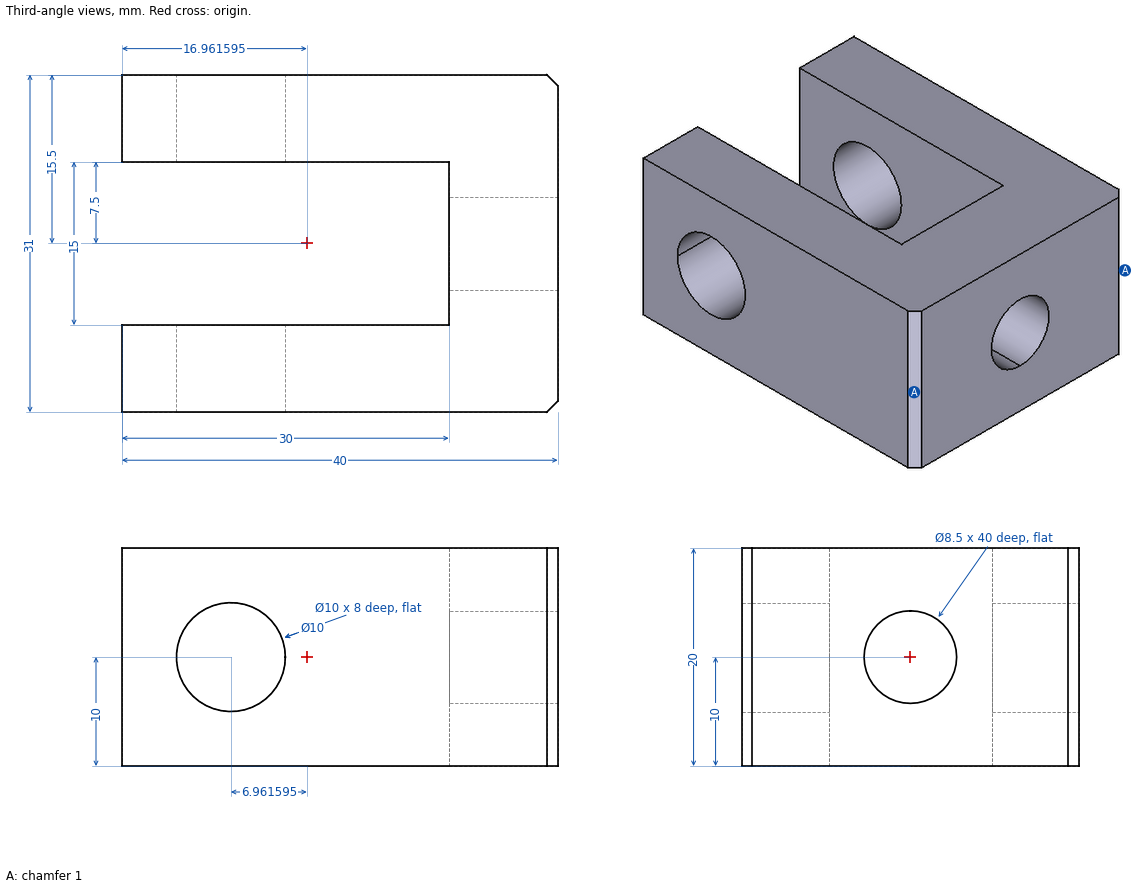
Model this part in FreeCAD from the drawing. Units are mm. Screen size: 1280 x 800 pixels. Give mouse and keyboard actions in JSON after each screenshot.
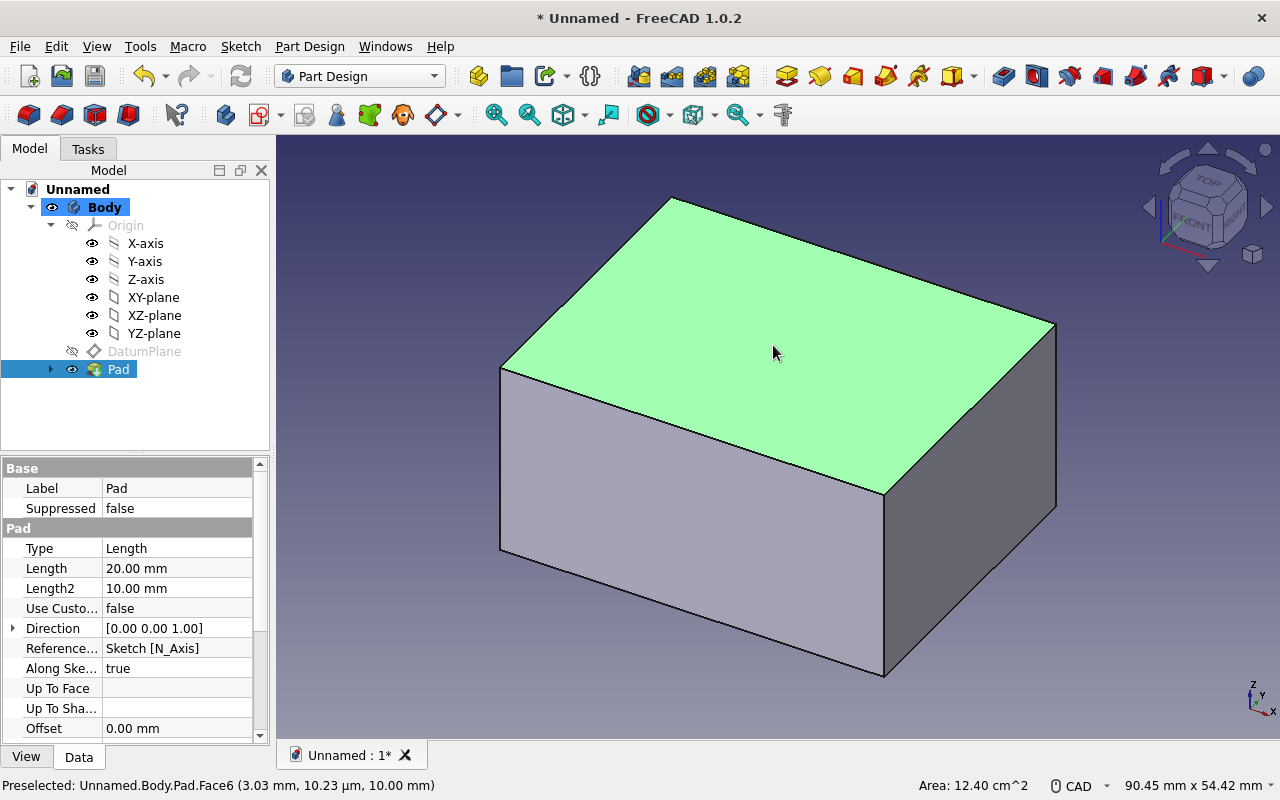
{"action": "left_click", "coordinate": [258, 116]}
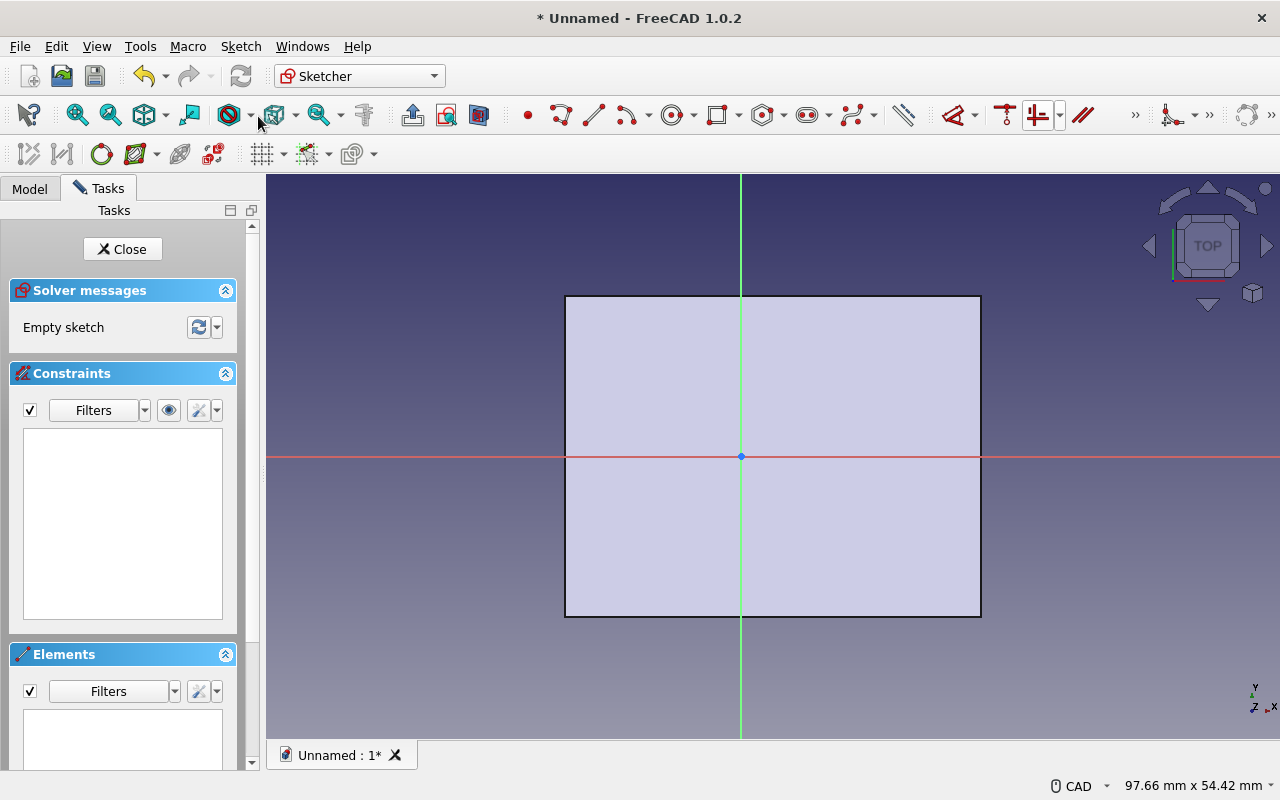
{"action": "scroll", "coordinate": [741, 456], "scroll_direction": "up", "scroll_amount": 3}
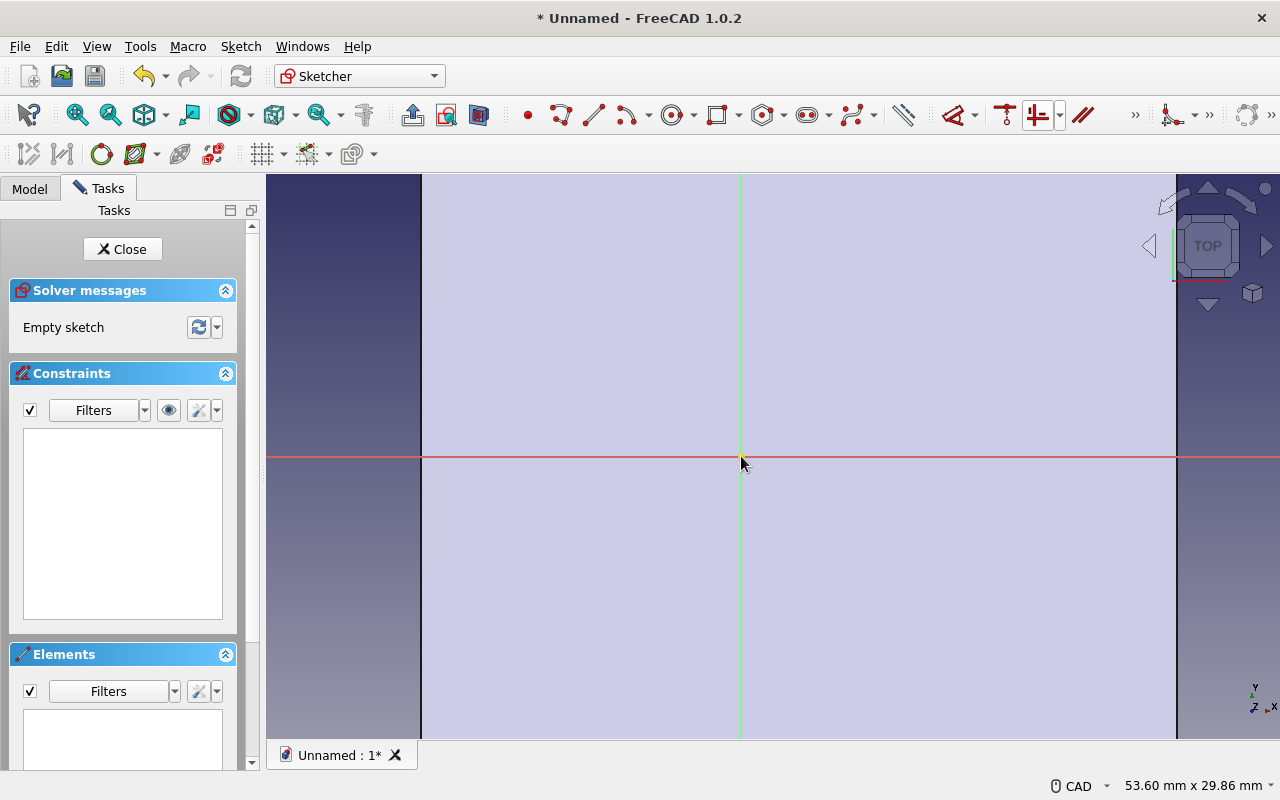
{"action": "key", "text": "g r"}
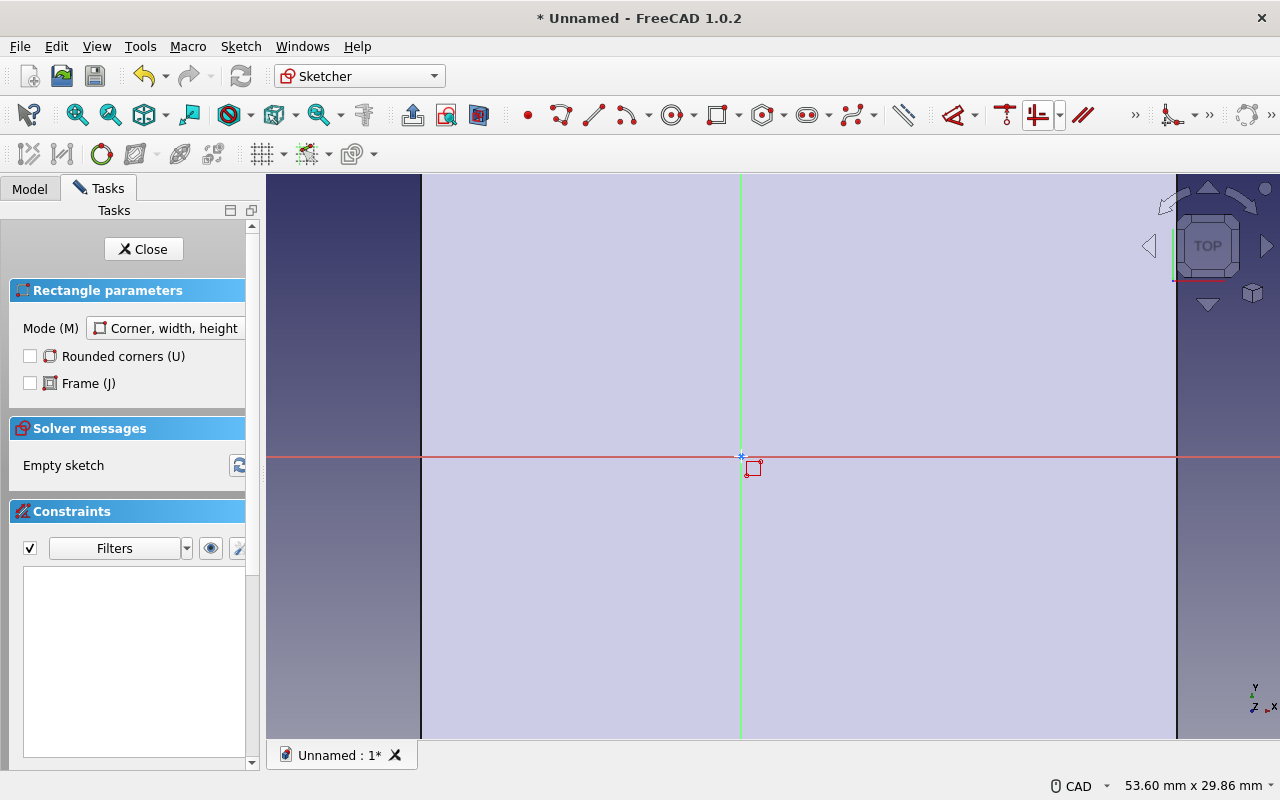
{"action": "left_click", "coordinate": [421, 315]}
{"action": "left_click", "coordinate": [988, 598]}
{"action": "key", "text": "Escape"}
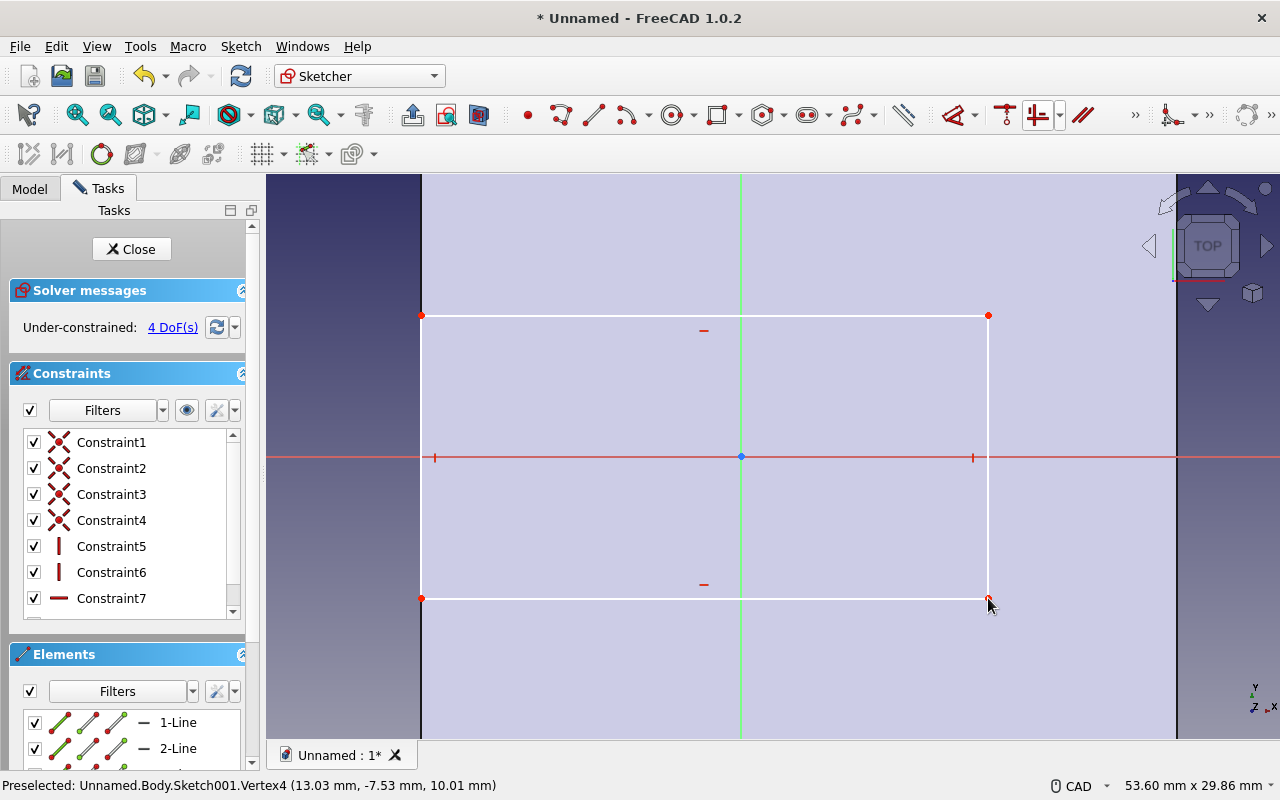
{"action": "key", "text": "d"}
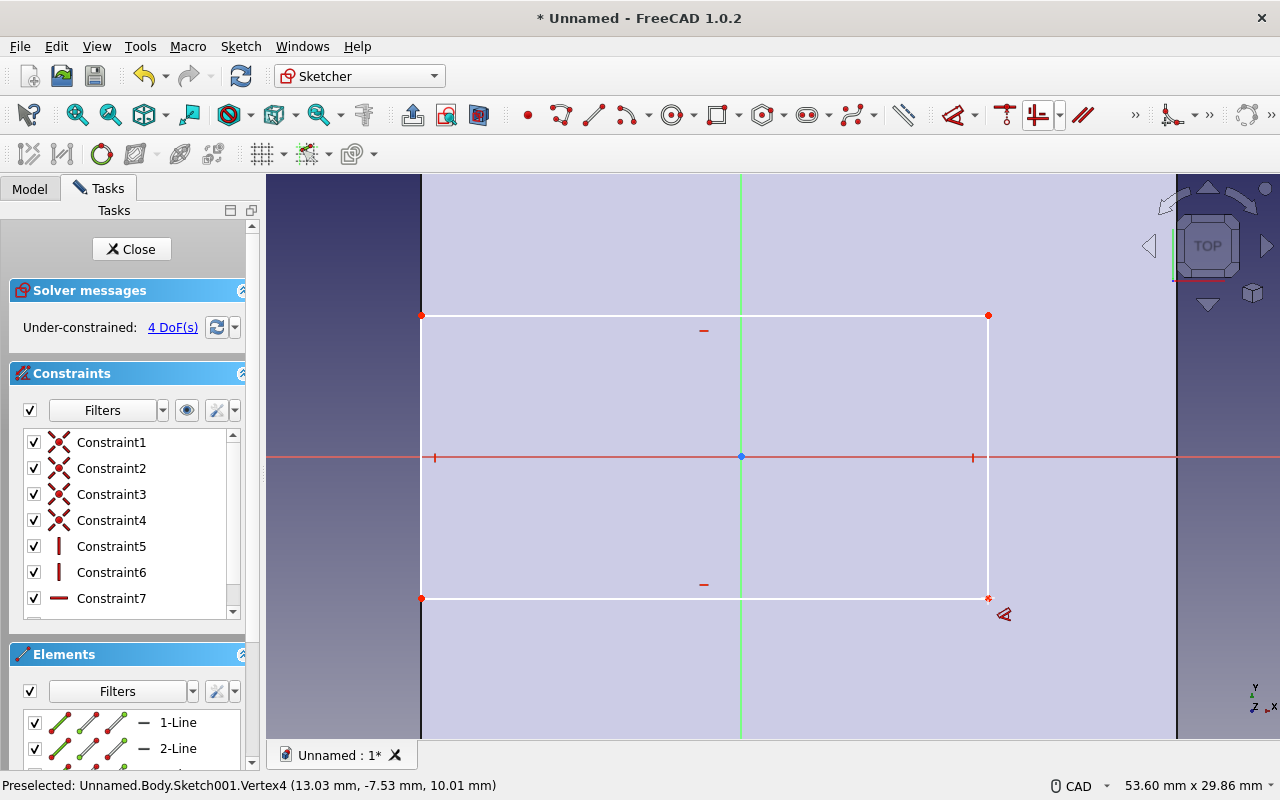
{"action": "left_click", "coordinate": [421, 401]}
{"action": "left_click", "coordinate": [387, 392]}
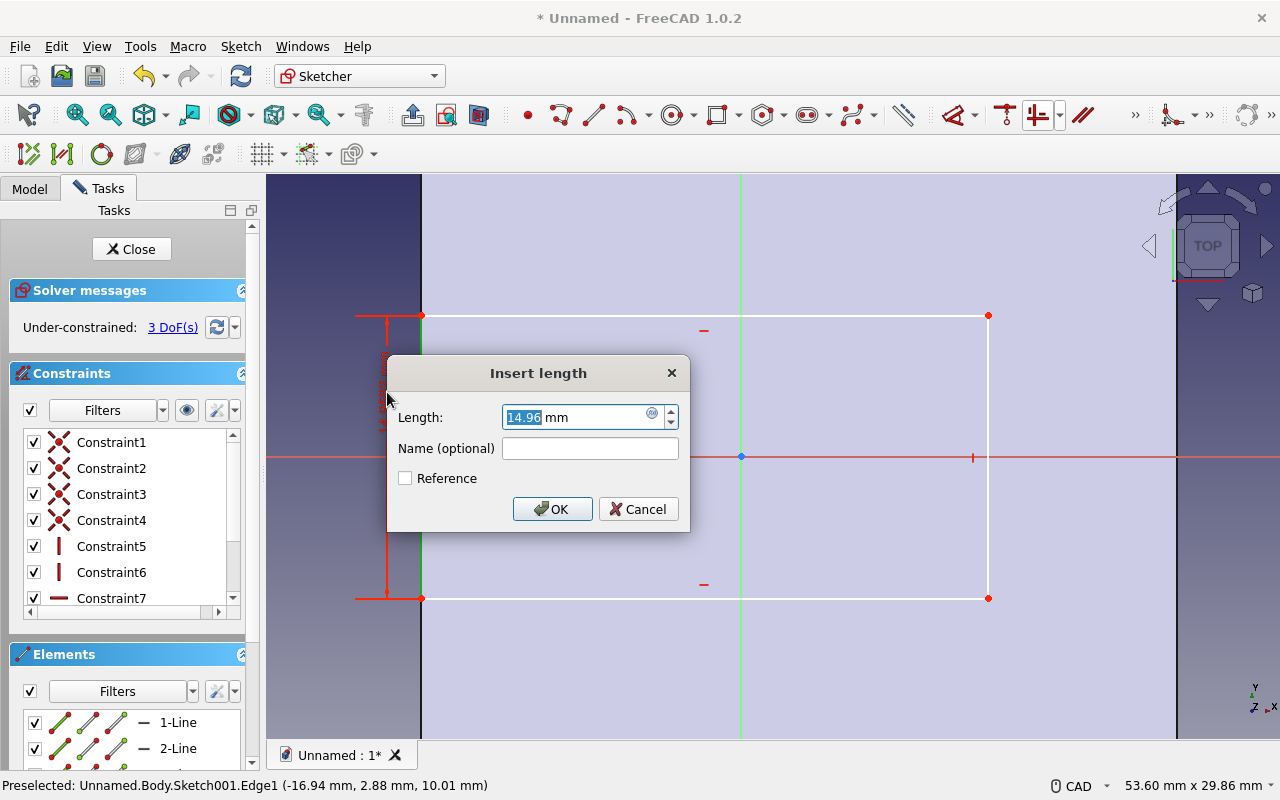
{"action": "type", "text": "15"}
{"action": "key", "text": "Return"}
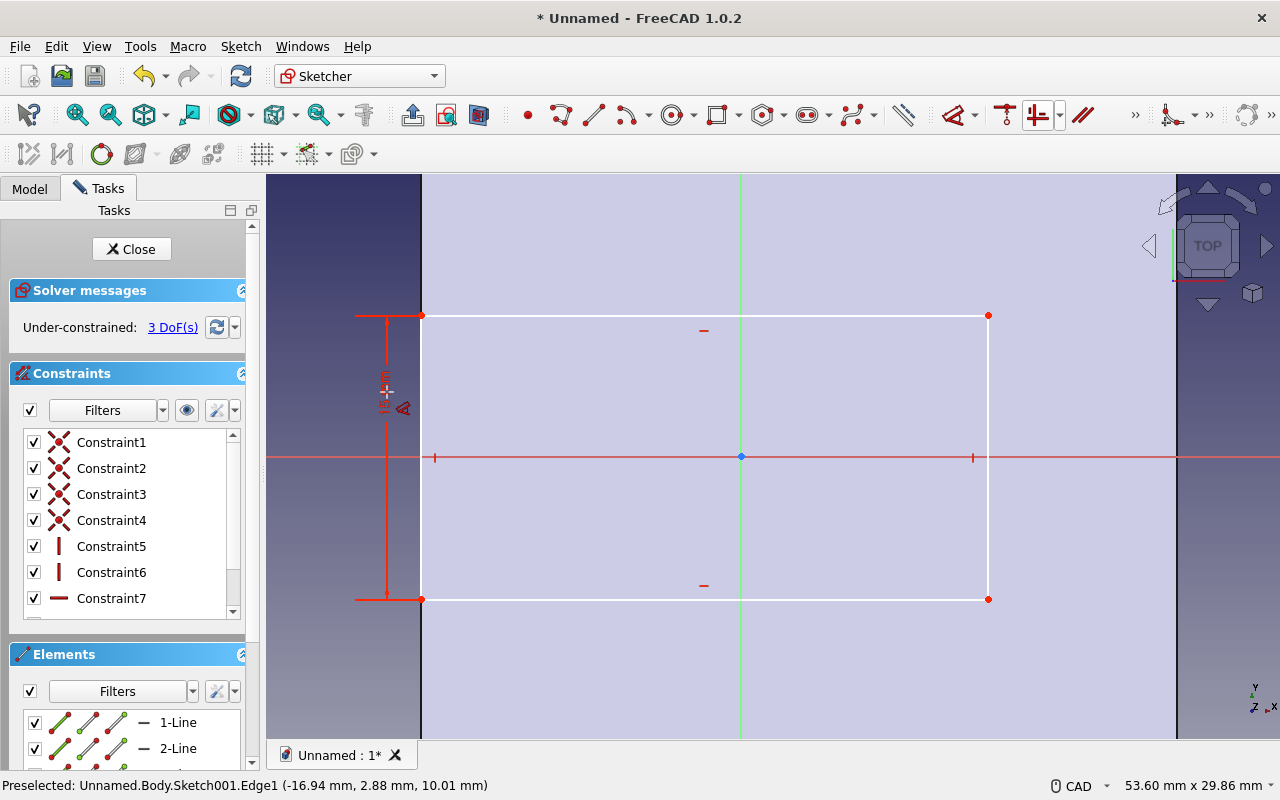
{"action": "left_click", "coordinate": [591, 600]}
{"action": "left_click", "coordinate": [704, 634]}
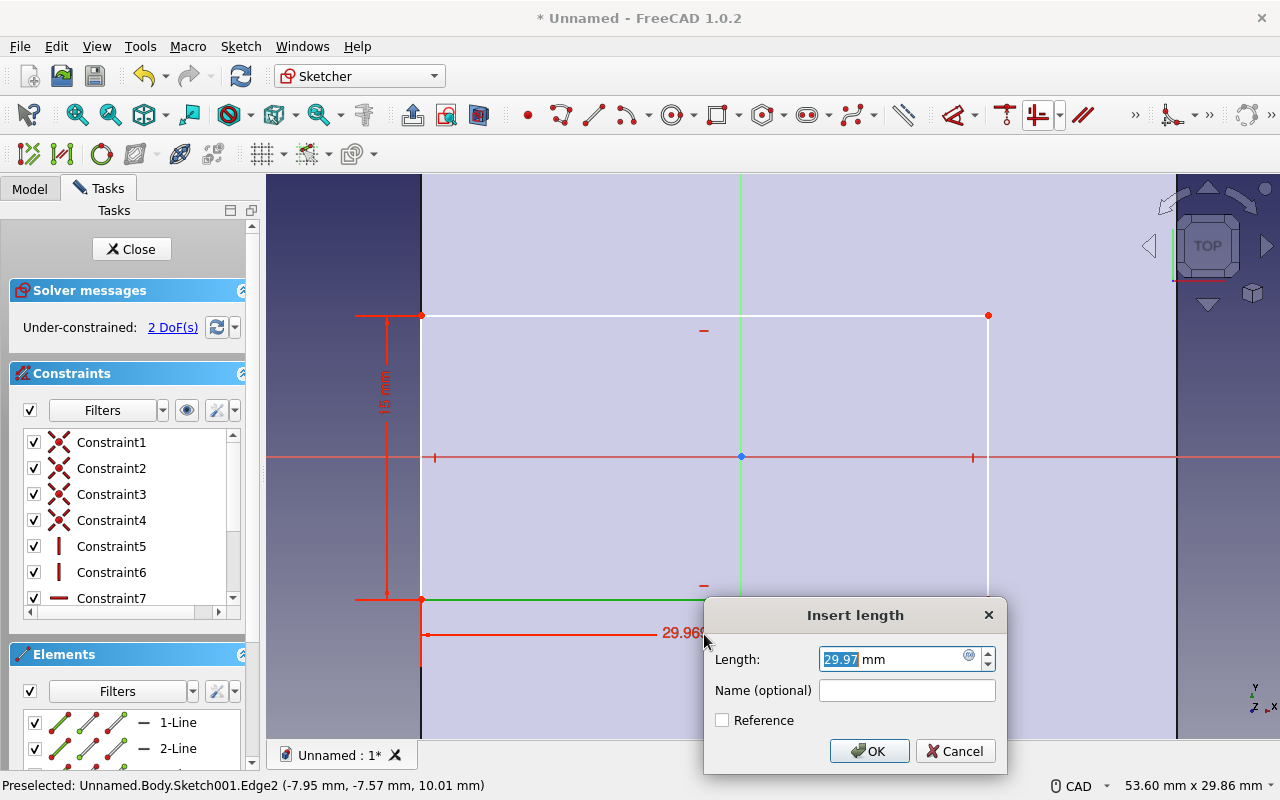
{"action": "type", "text": "30"}
{"action": "key", "text": "Return"}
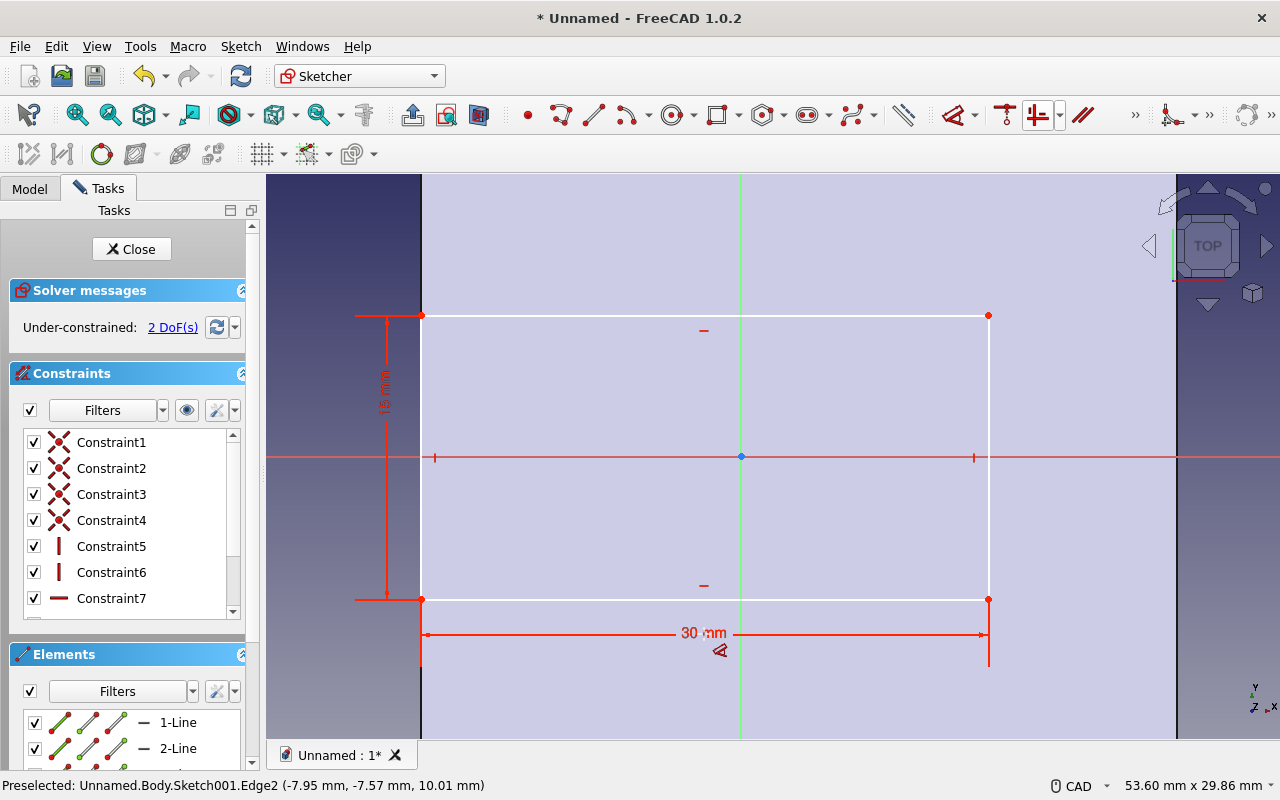
{"action": "left_click", "coordinate": [421, 316]}
{"action": "left_click", "coordinate": [387, 354]}